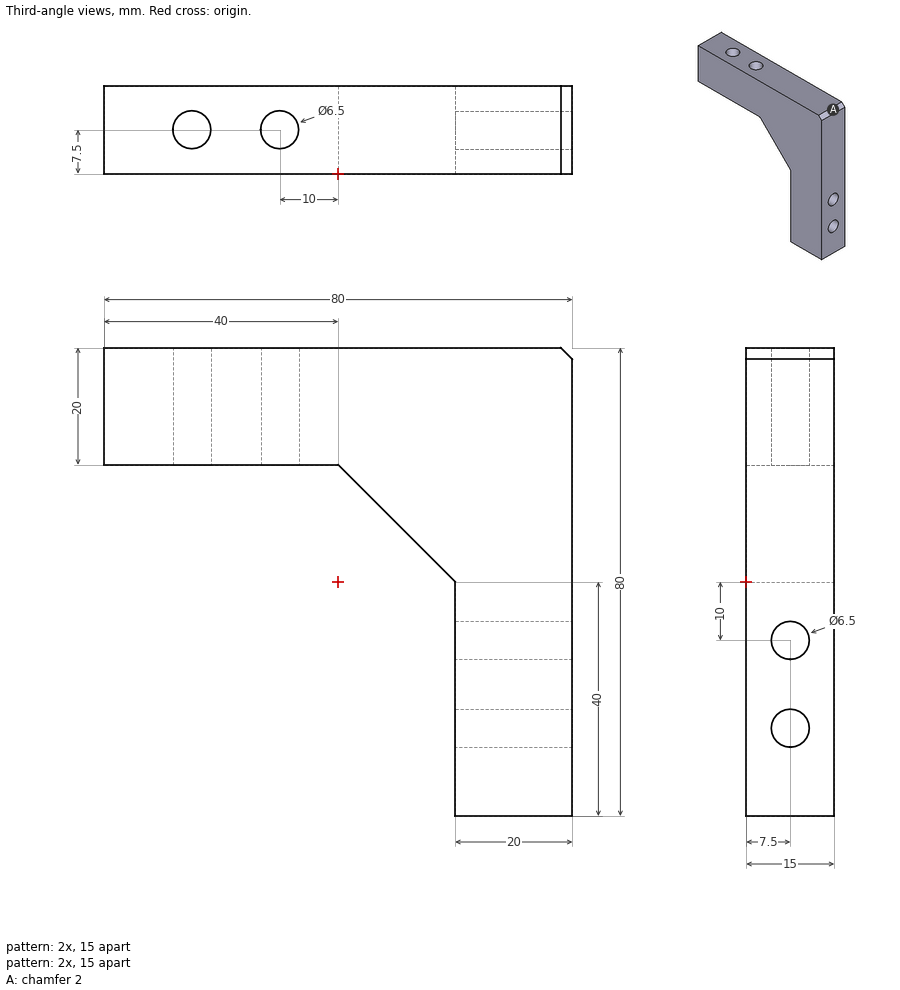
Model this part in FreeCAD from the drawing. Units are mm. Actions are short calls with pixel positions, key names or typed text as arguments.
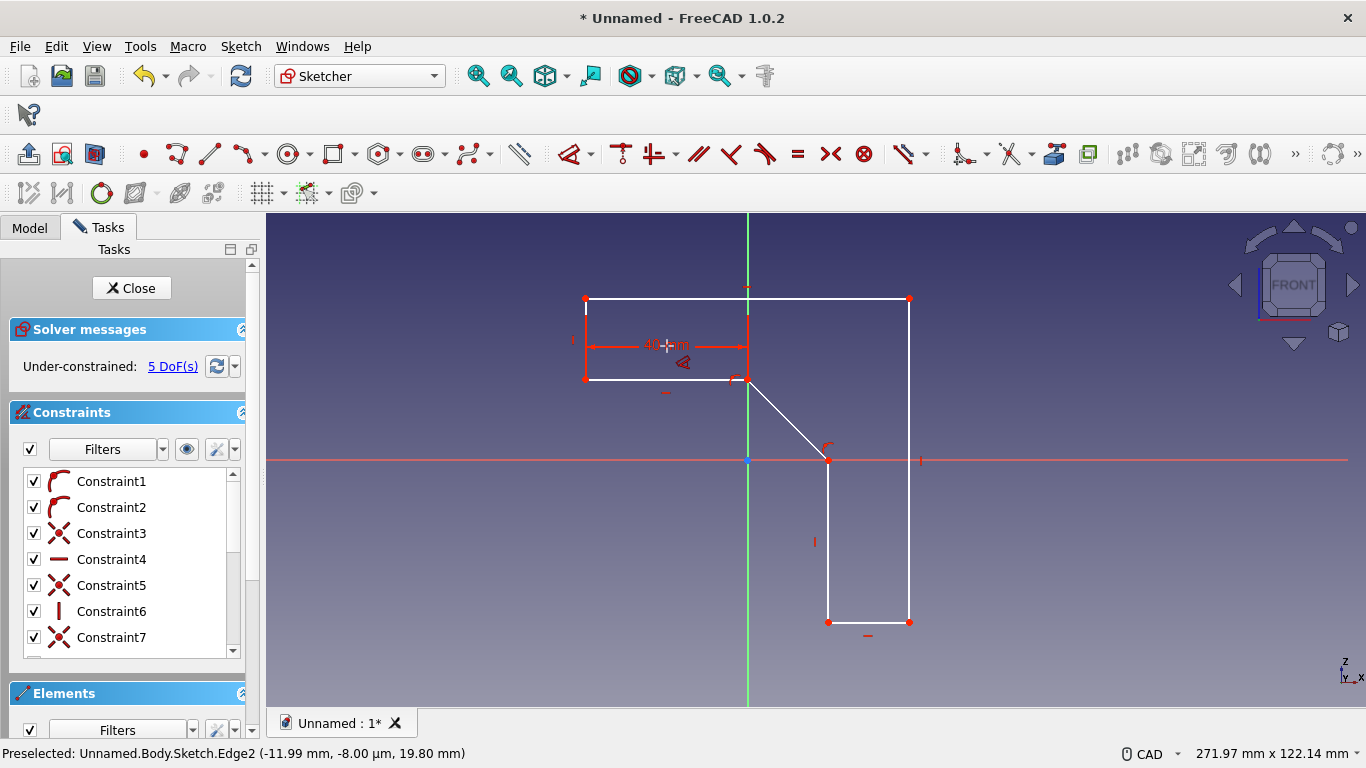
click(586, 356)
click(552, 340)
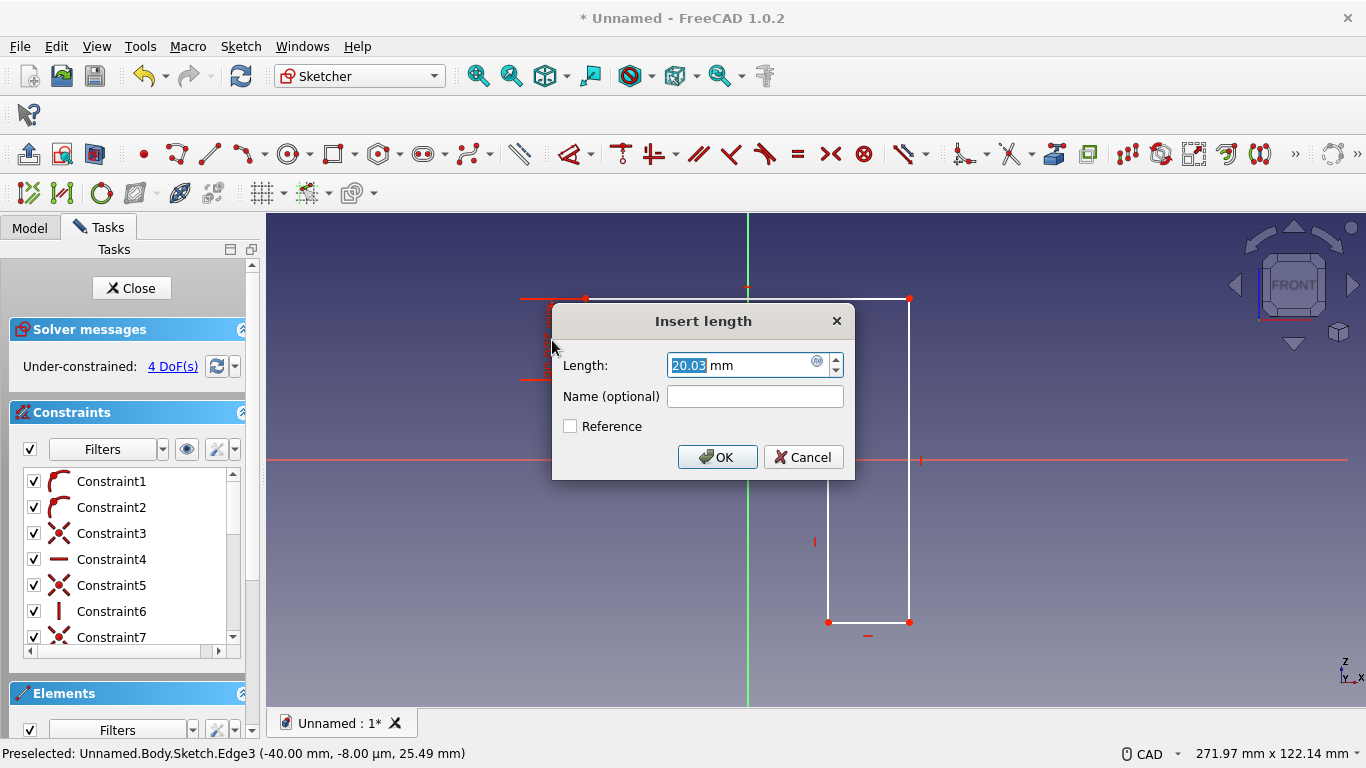
text(20)
key(Return)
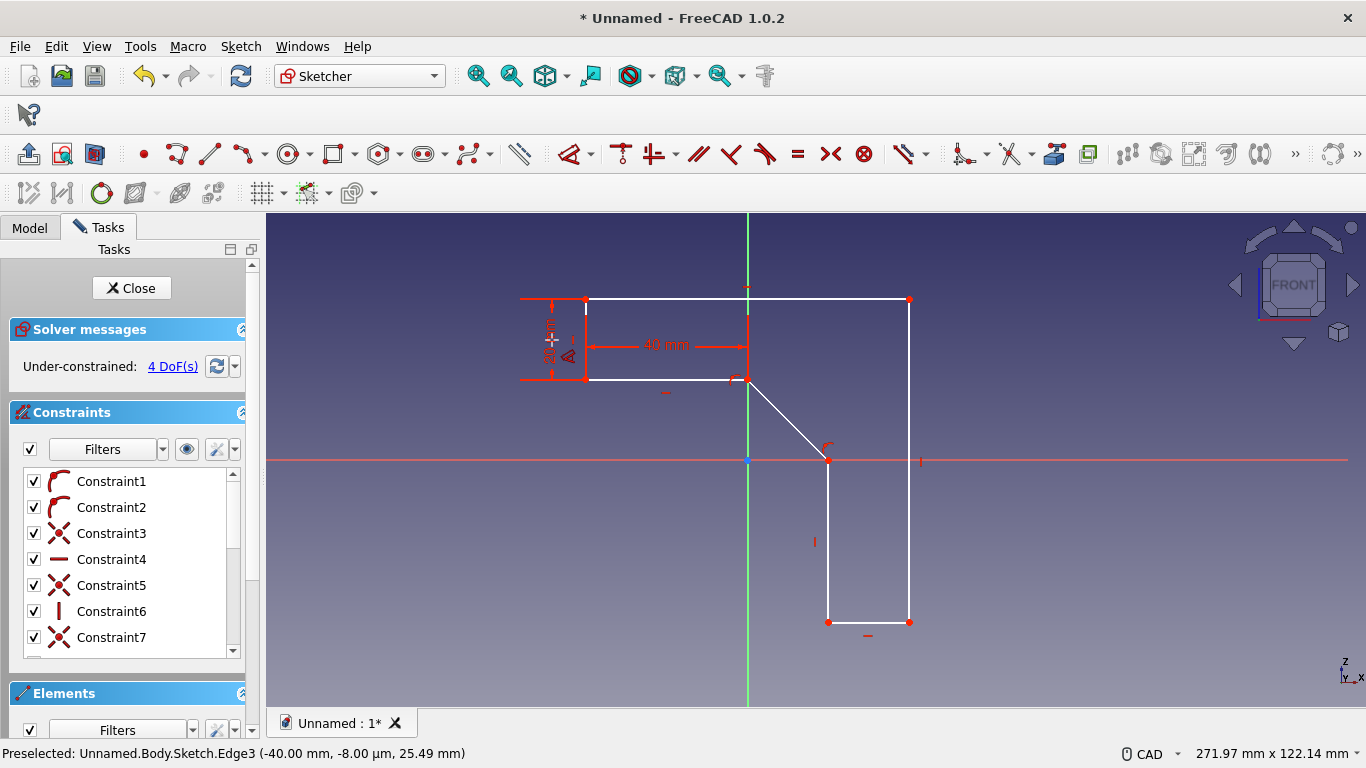
click(683, 299)
click(673, 265)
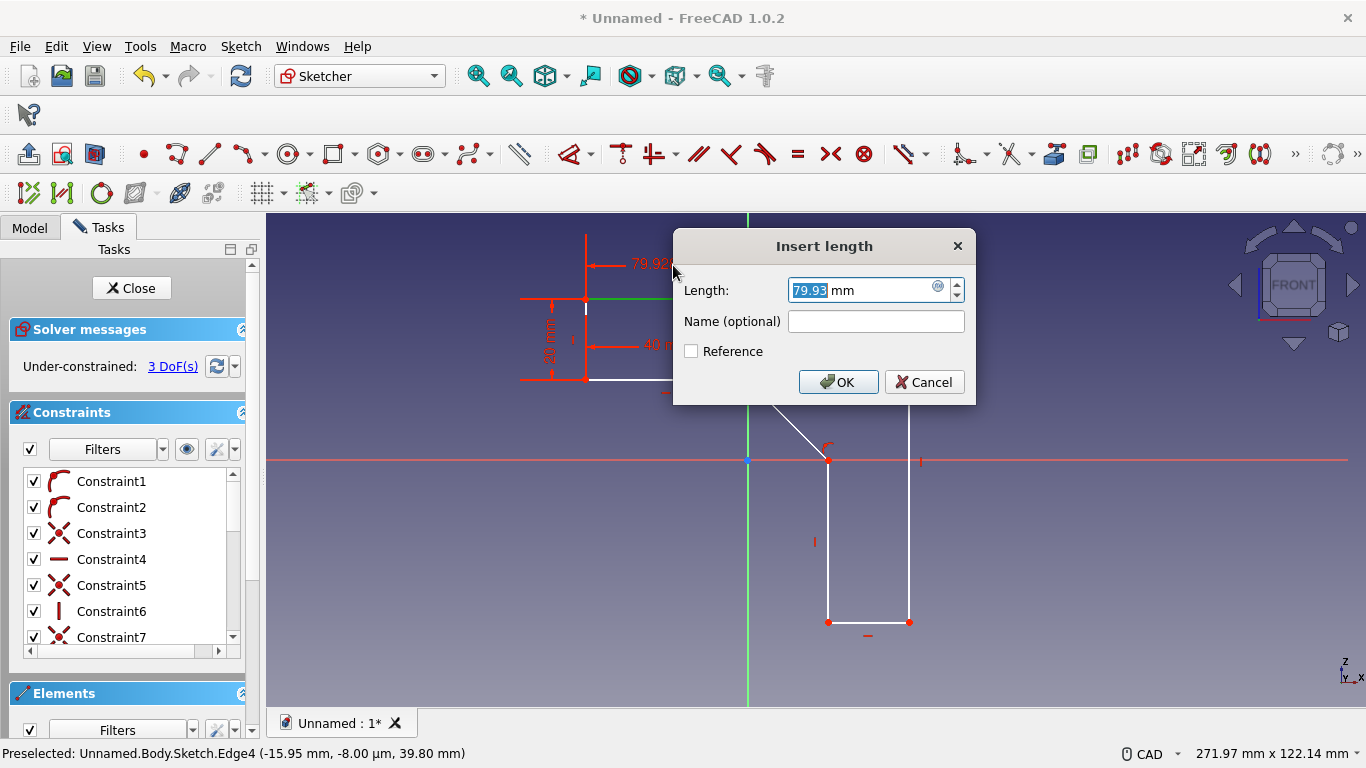
text(80)
key(Return)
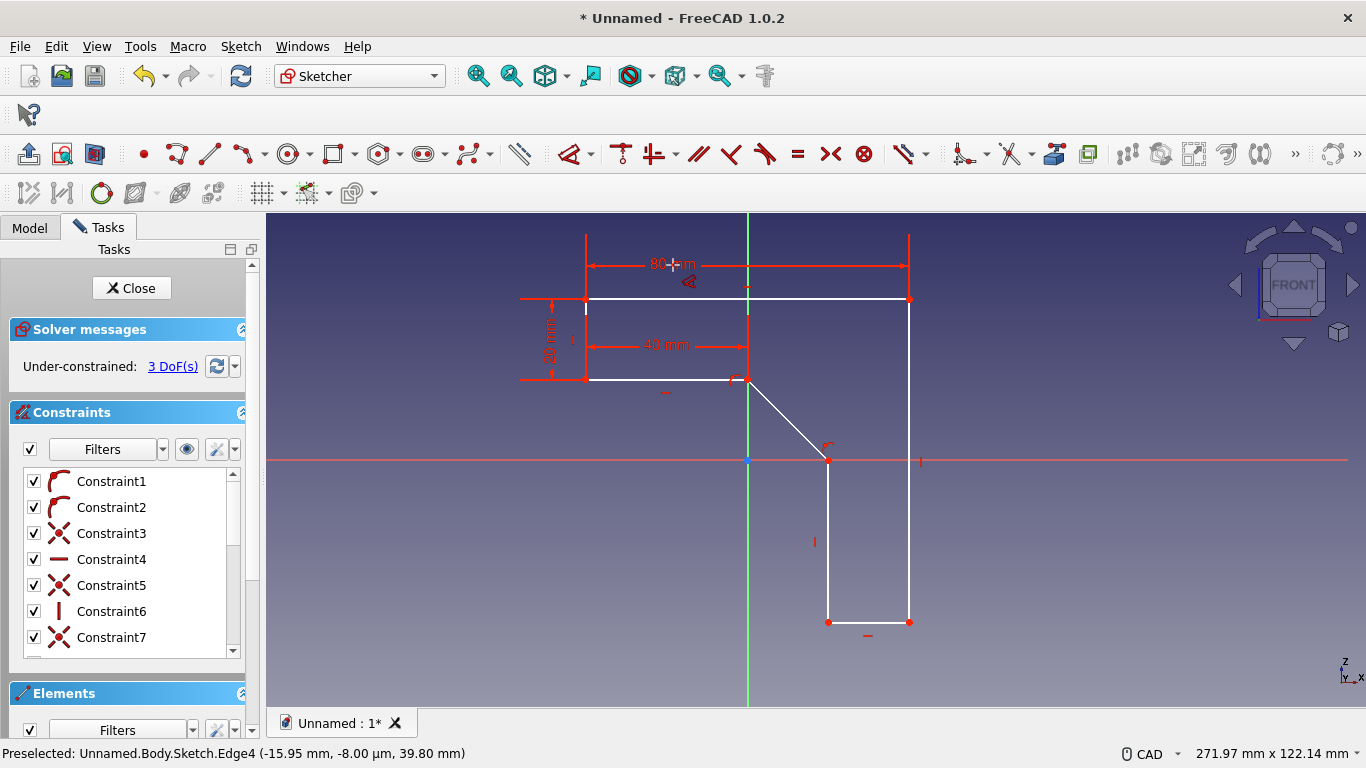
click(909, 396)
click(943, 387)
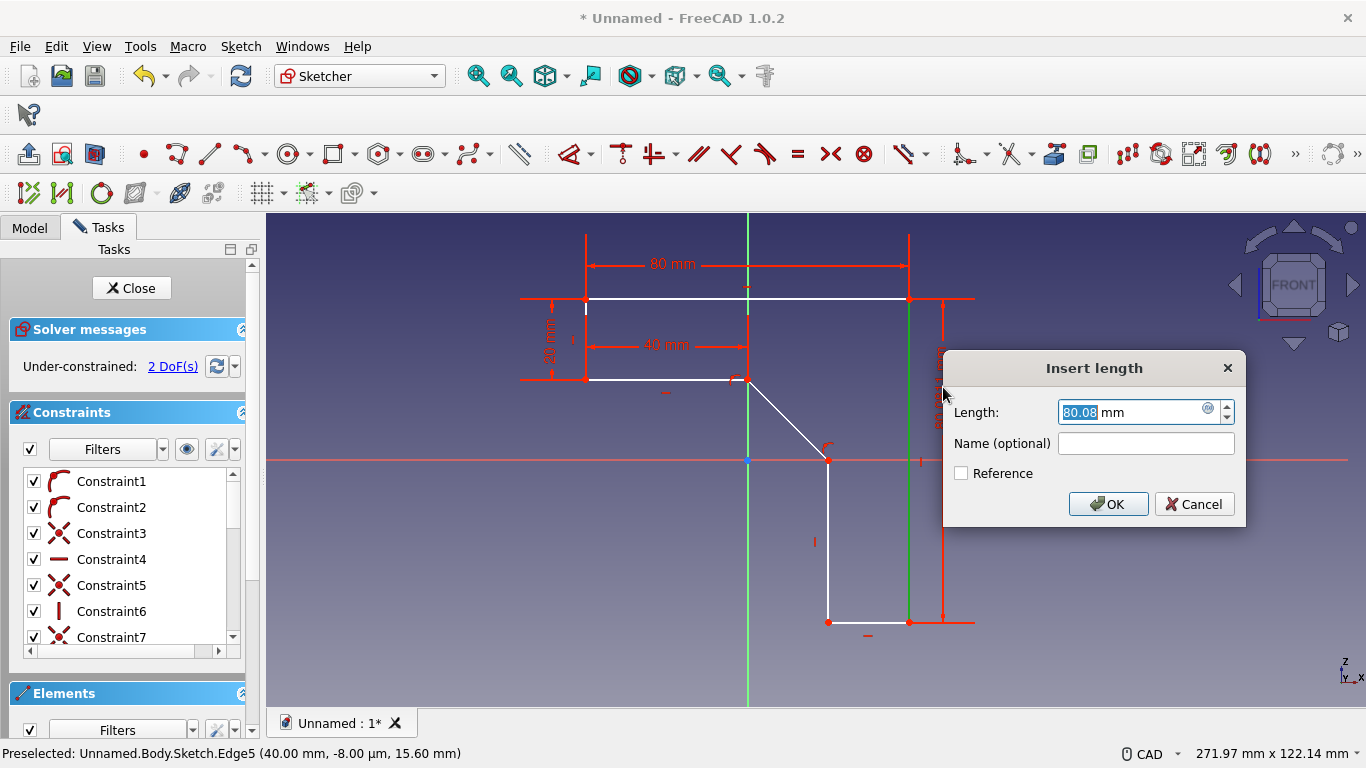
text(80)
key(Return)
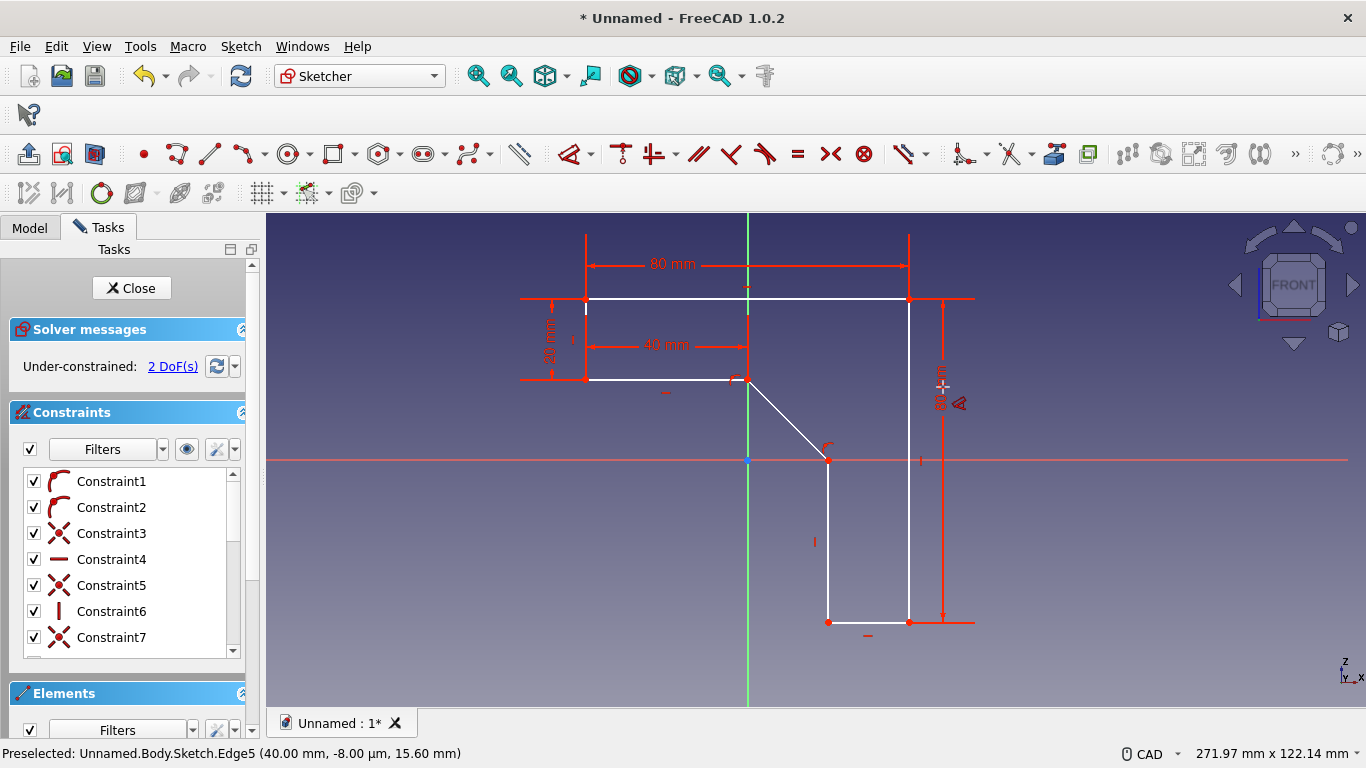
click(885, 623)
click(869, 657)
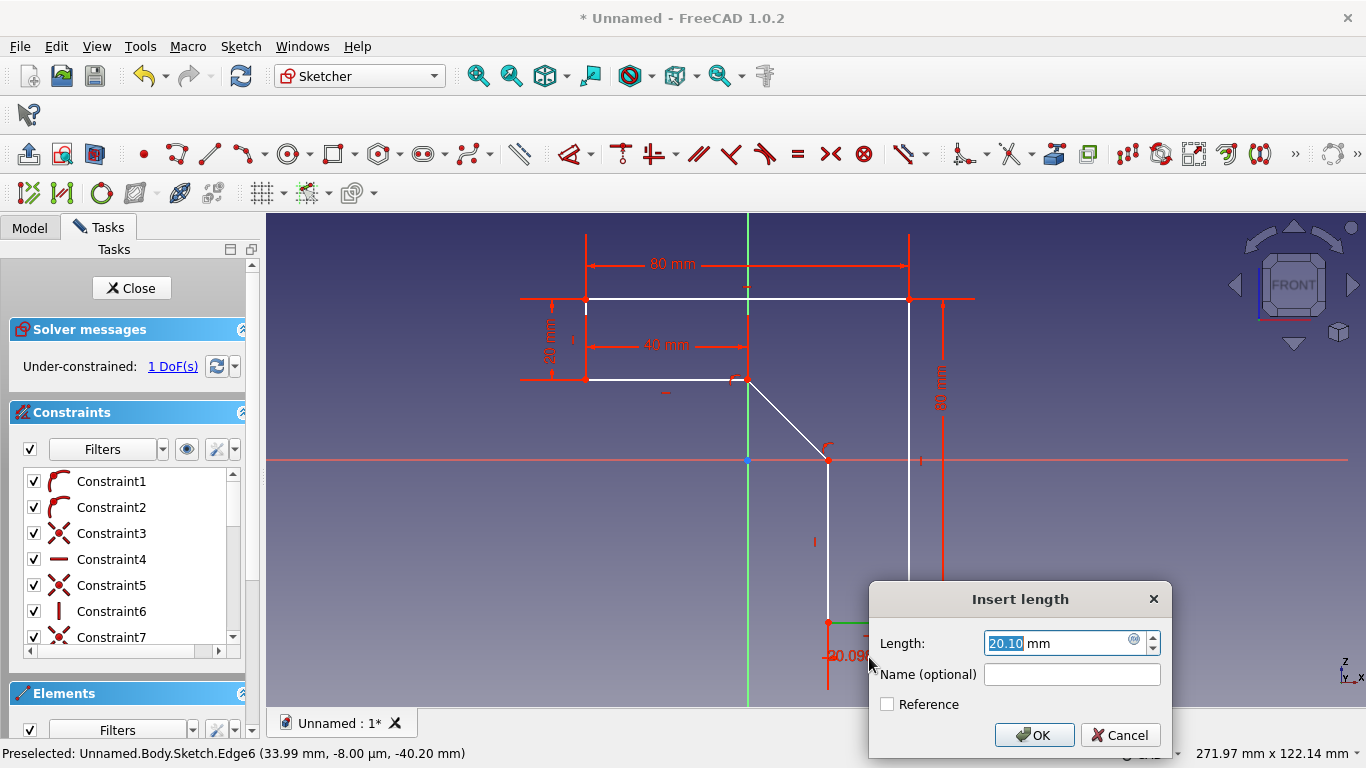
text(20)
key(Return)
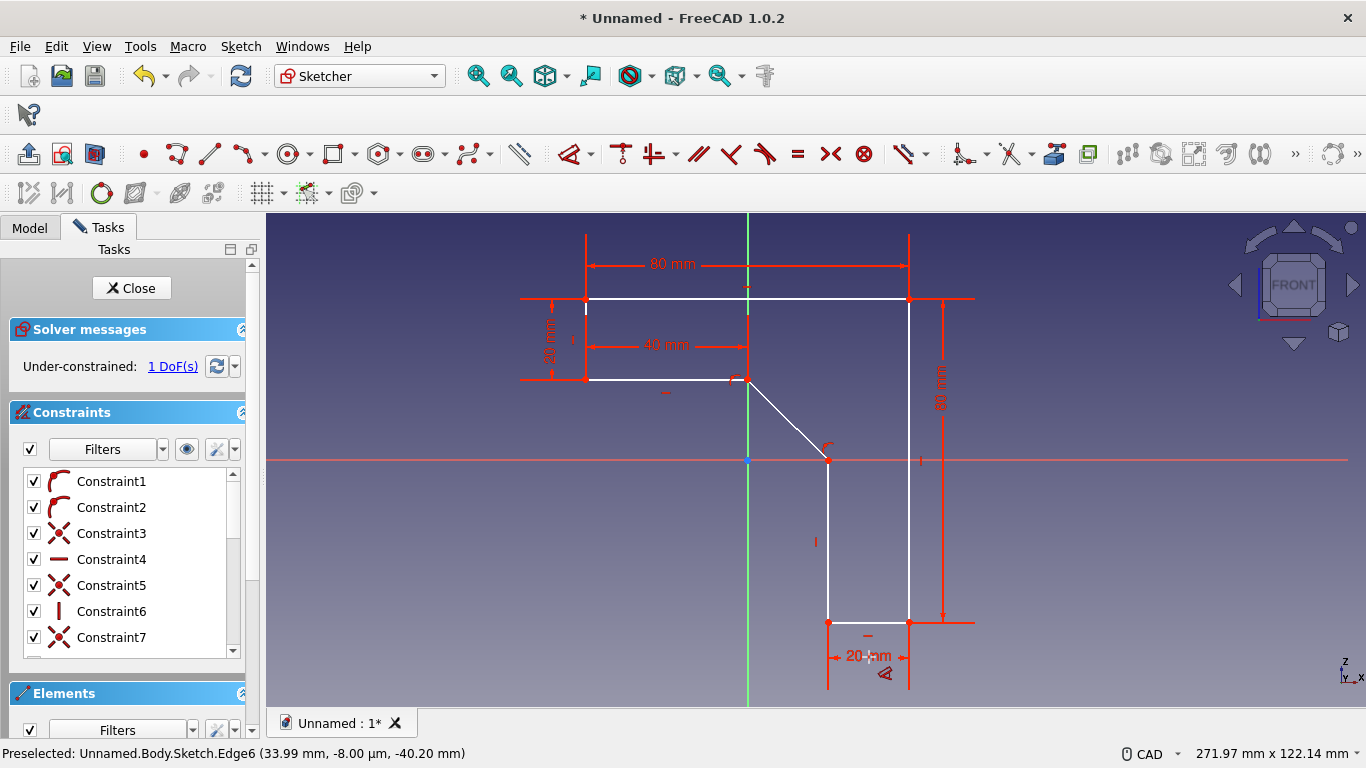
click(828, 574)
click(862, 541)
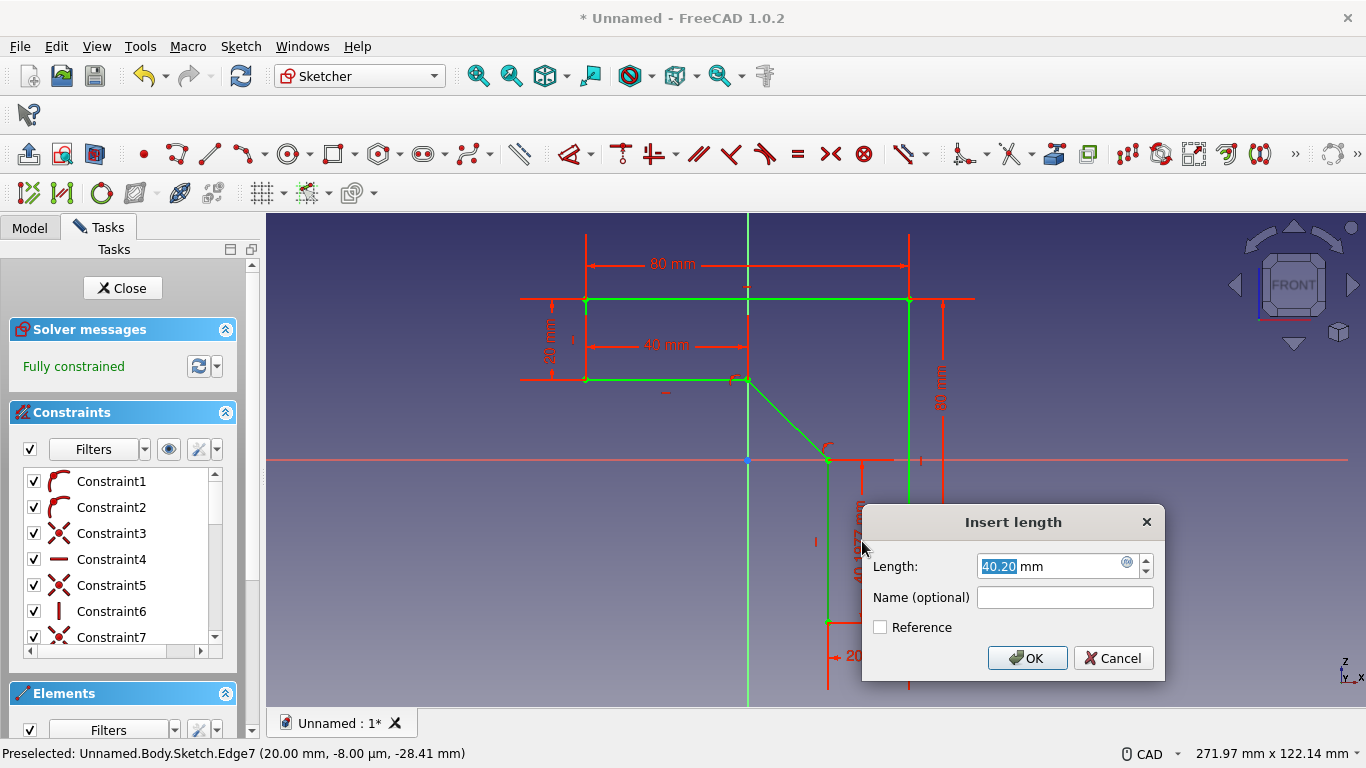
text(40)
key(Return)
key(Escape)